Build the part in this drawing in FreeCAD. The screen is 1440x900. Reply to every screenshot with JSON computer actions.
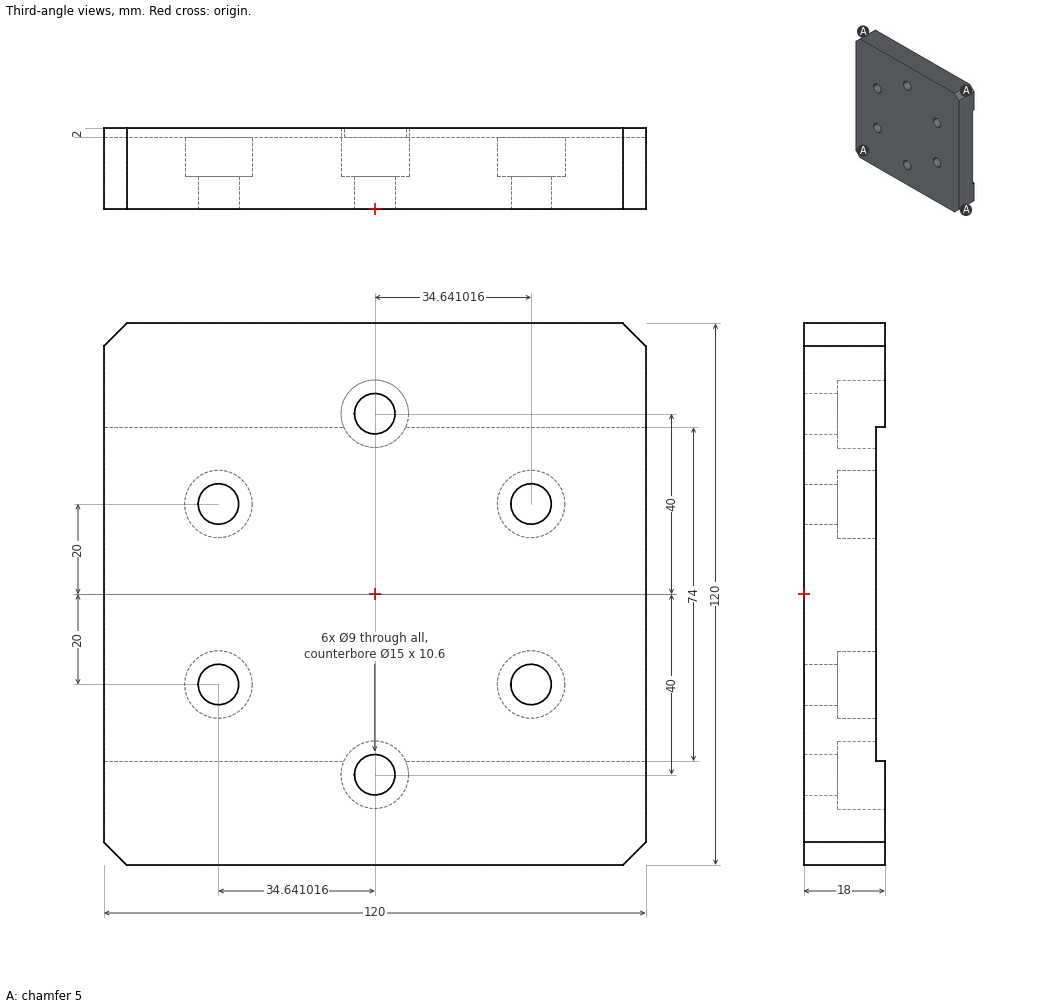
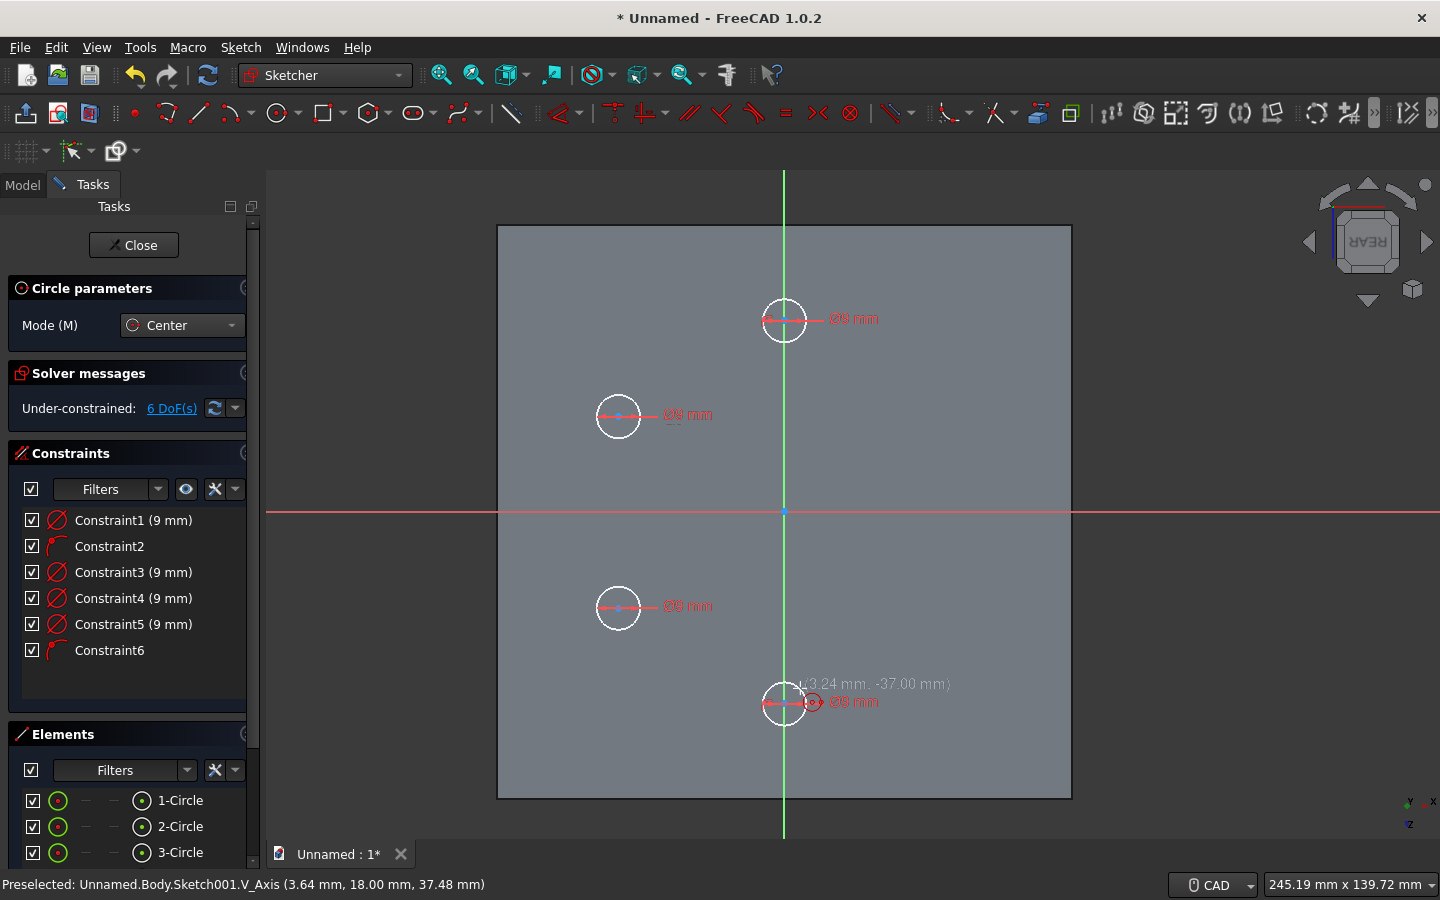
{"action": "left_click", "coordinate": [950, 608]}
{"action": "mouse_move", "coordinate": [966, 592]}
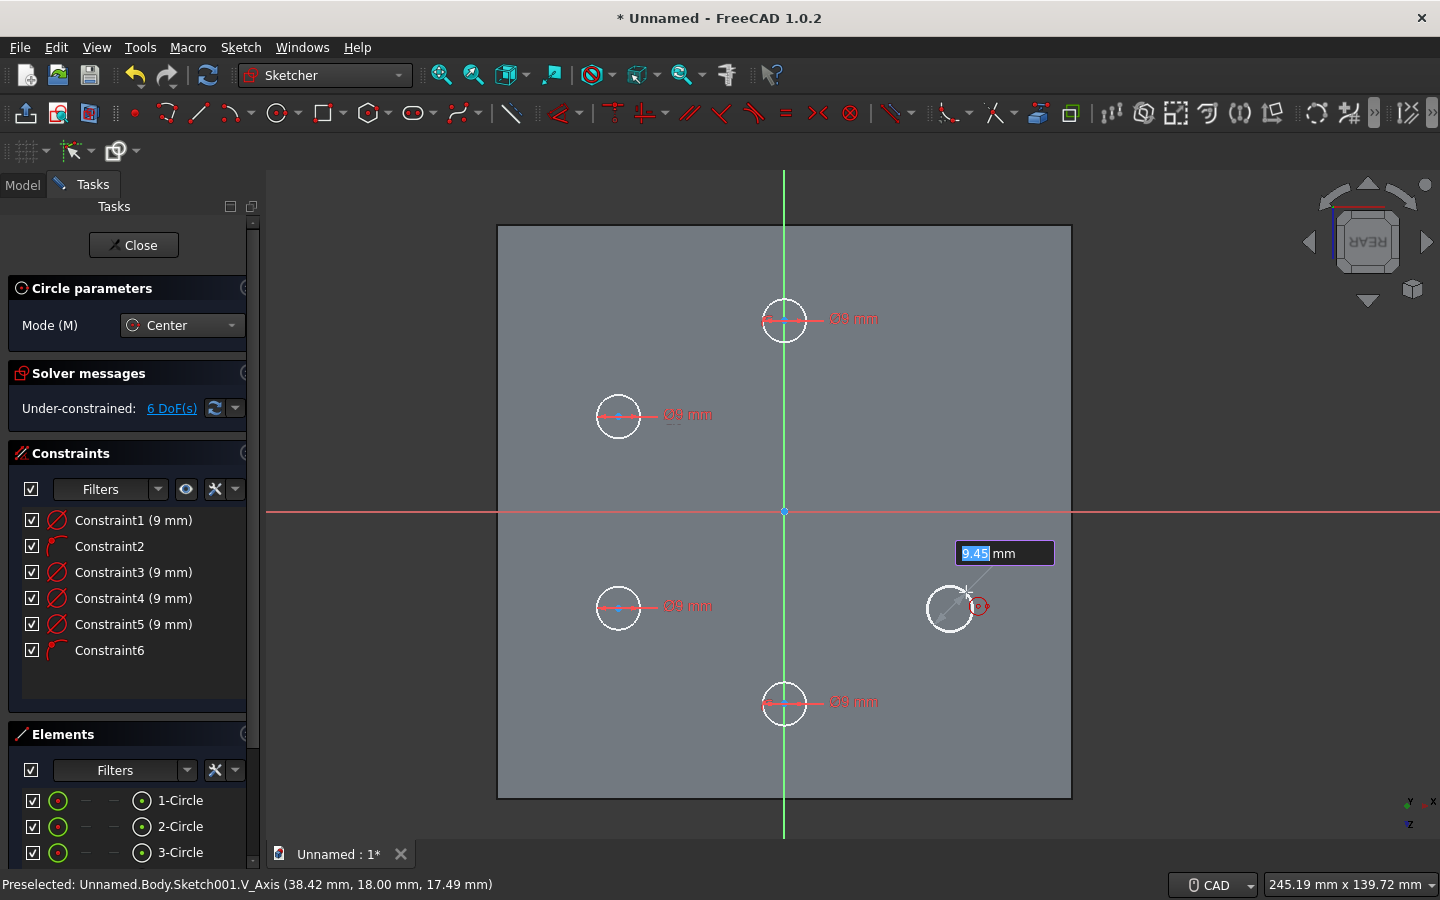
{"action": "type", "text": "9"}
{"action": "key", "text": "Return"}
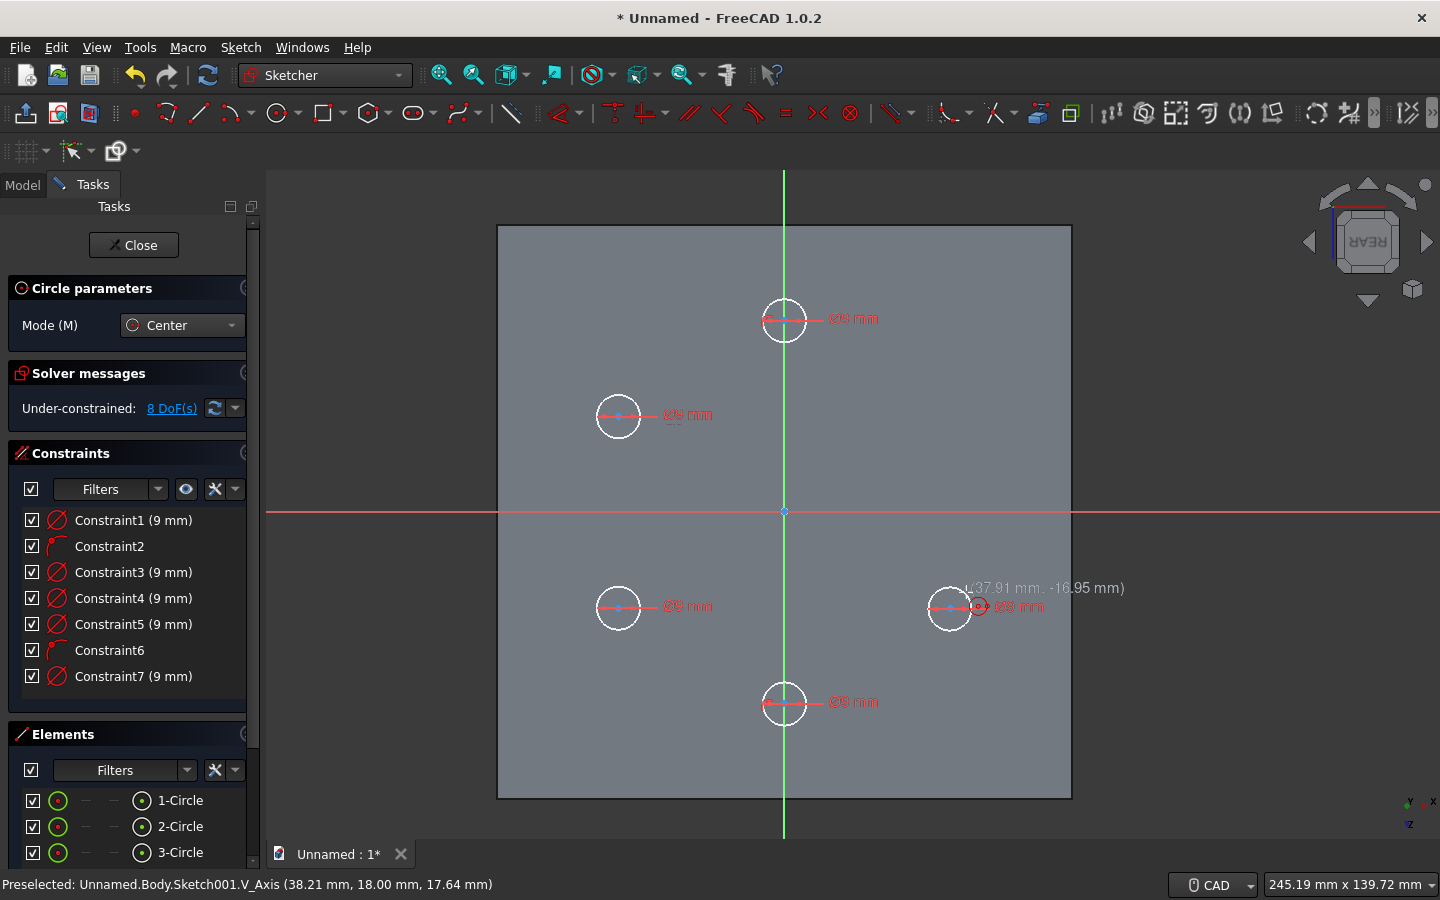
{"action": "left_click", "coordinate": [950, 416]}
{"action": "mouse_move", "coordinate": [966, 401]}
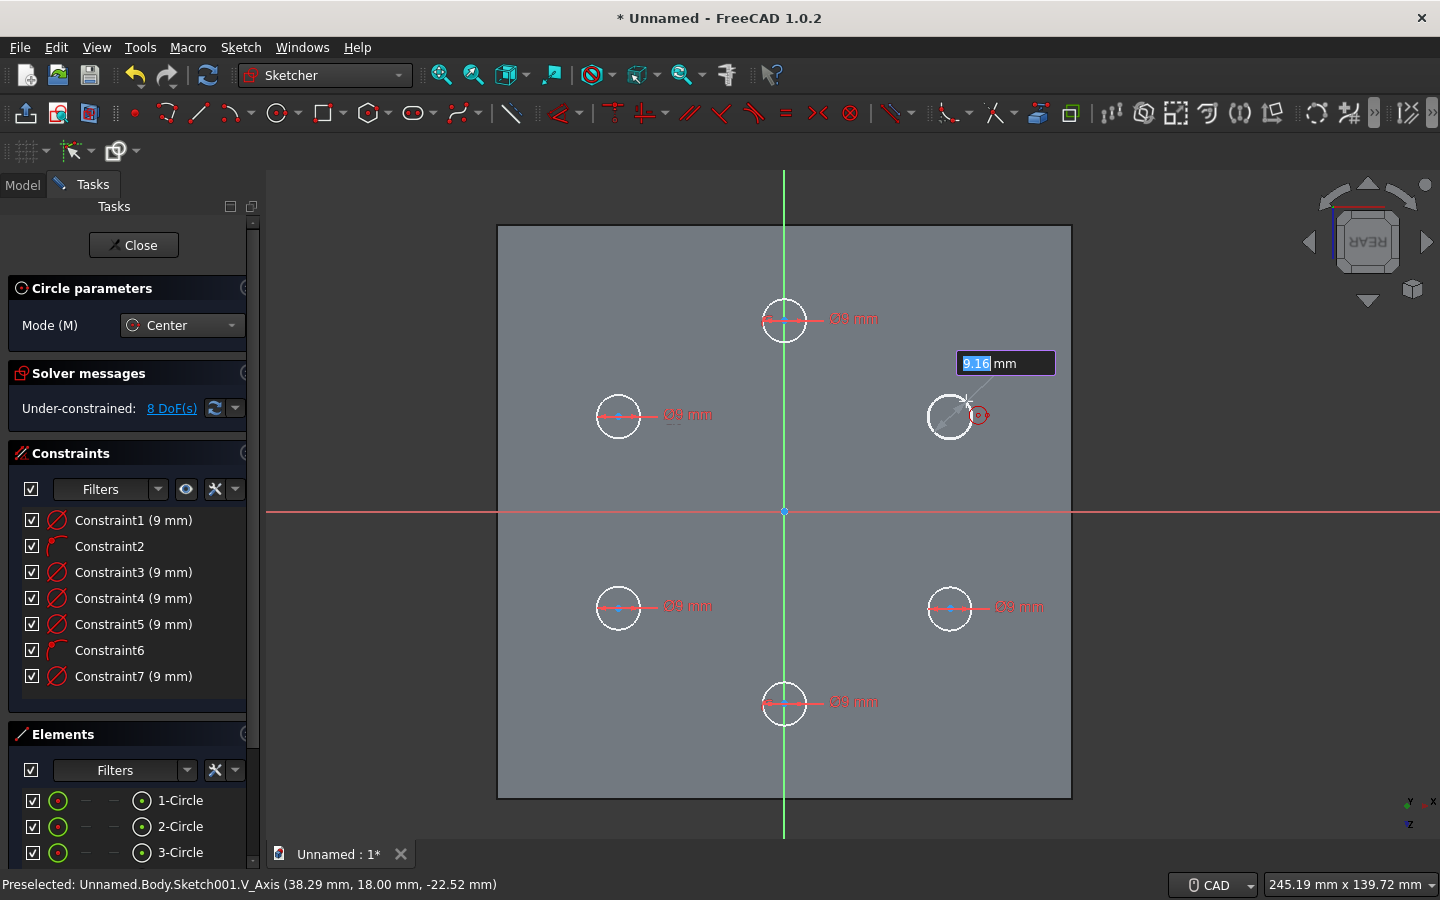
{"action": "type", "text": "9"}
{"action": "key", "text": "Return"}
{"action": "key", "text": "Escape"}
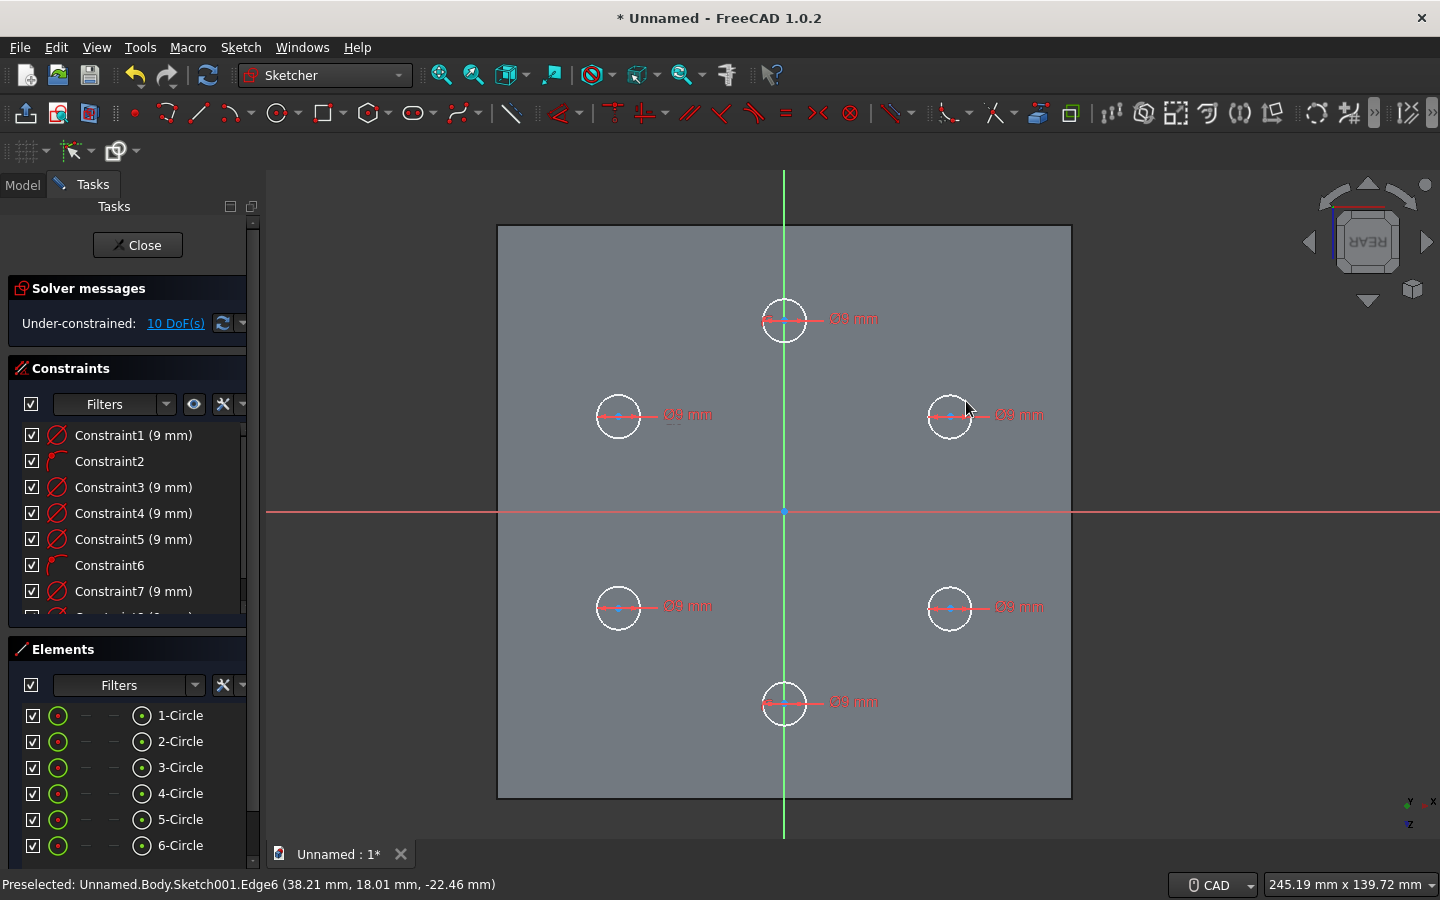
{"action": "left_click", "coordinate": [618, 417]}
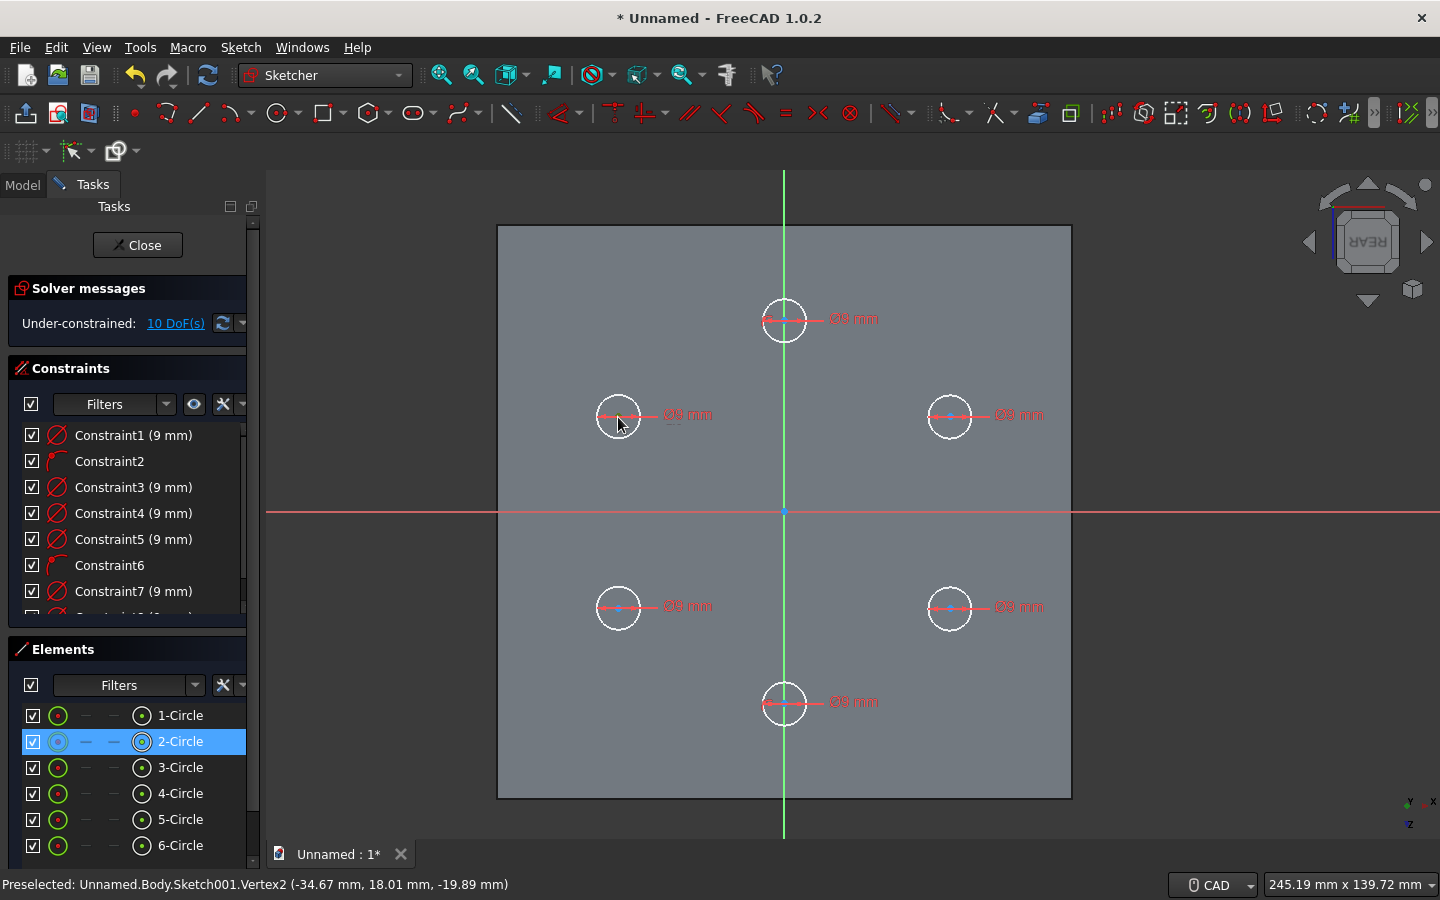
{"action": "left_click", "coordinate": [618, 608]}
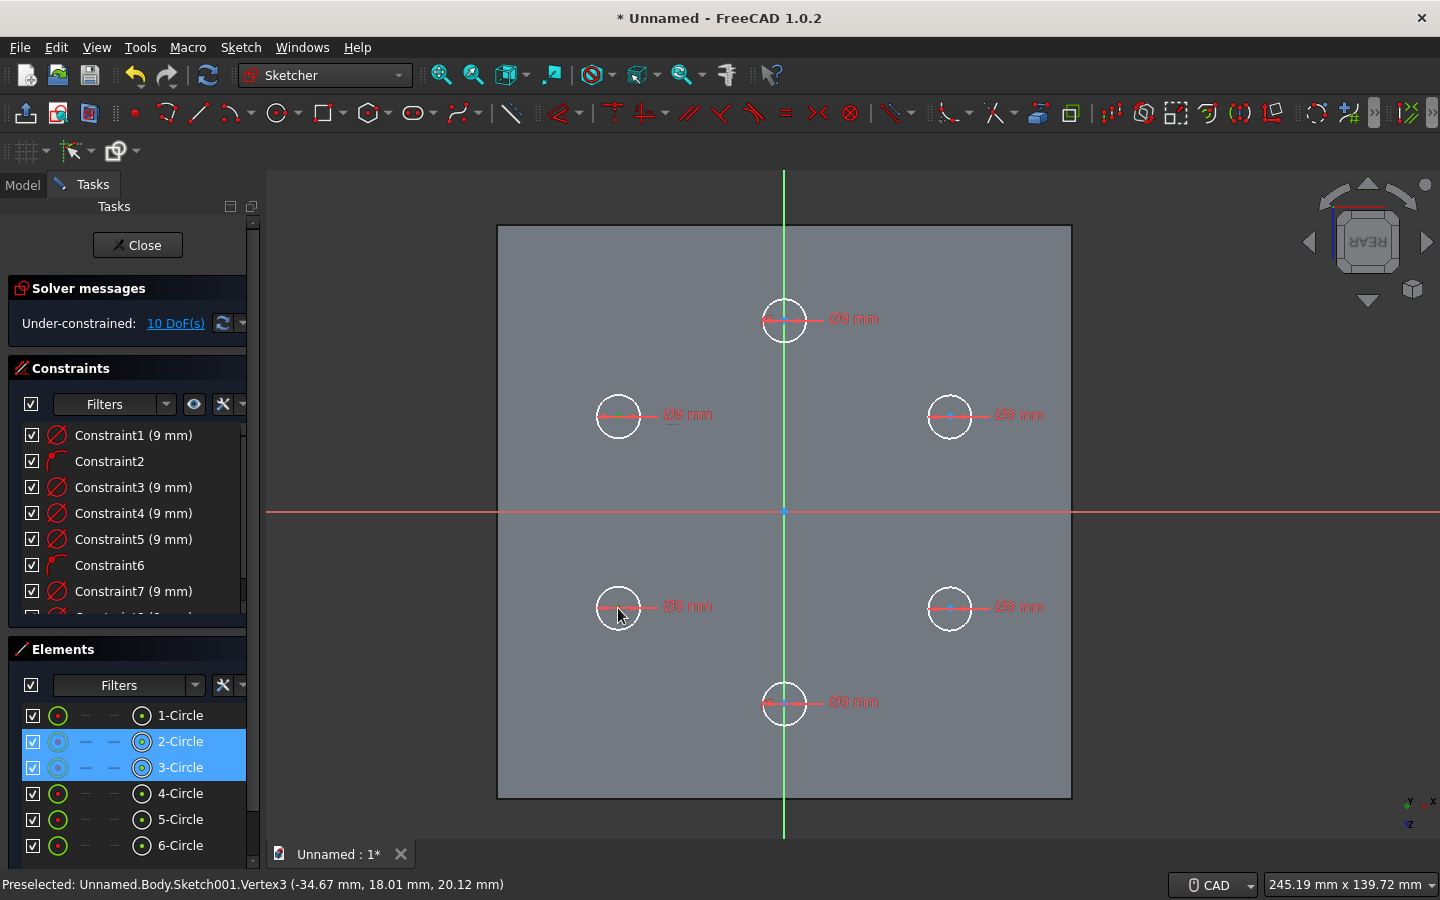
{"action": "key", "text": "v"}